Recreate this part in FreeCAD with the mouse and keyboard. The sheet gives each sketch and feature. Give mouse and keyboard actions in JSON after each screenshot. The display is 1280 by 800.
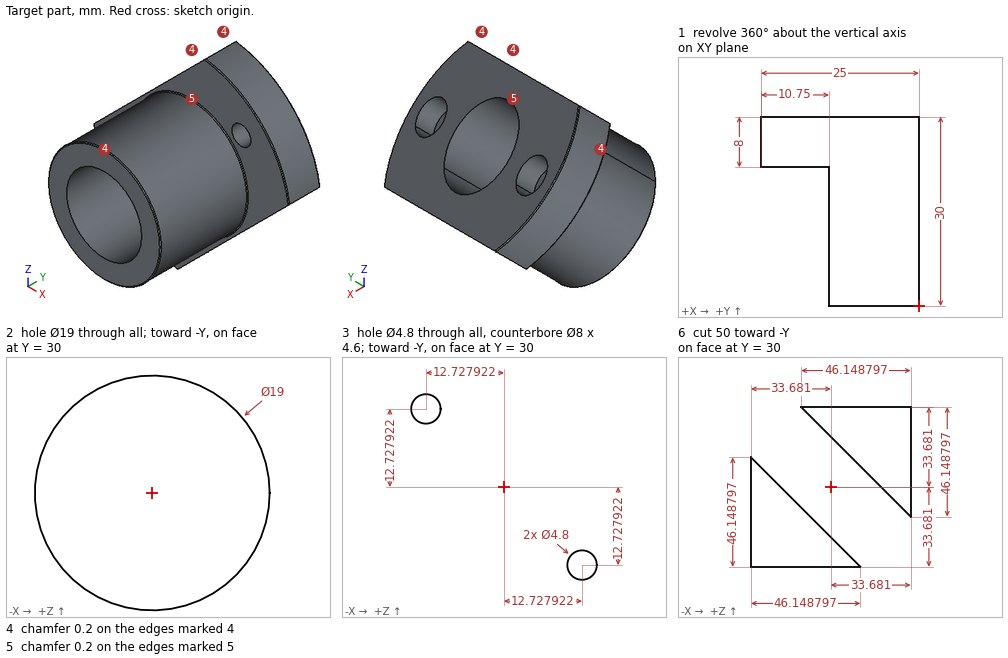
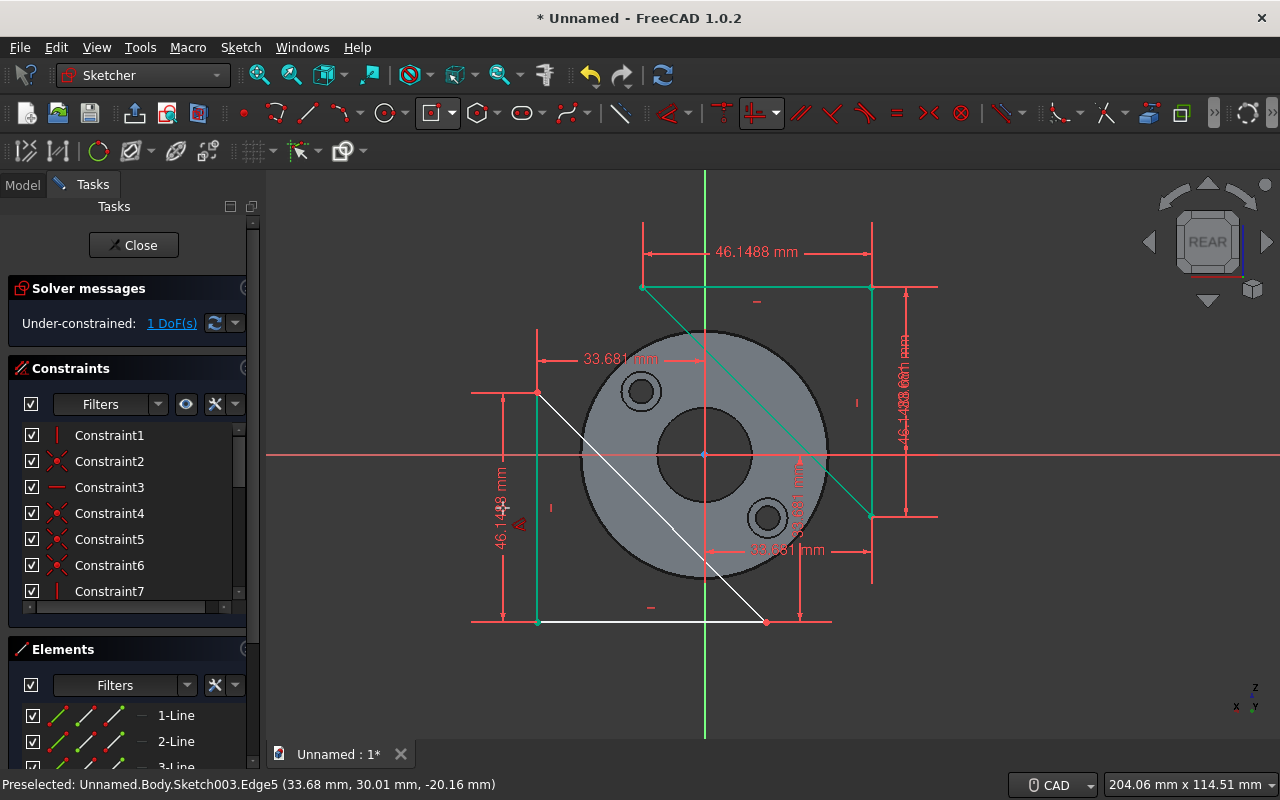
{"action": "left_click", "coordinate": [606, 622]}
{"action": "left_click", "coordinate": [652, 656]}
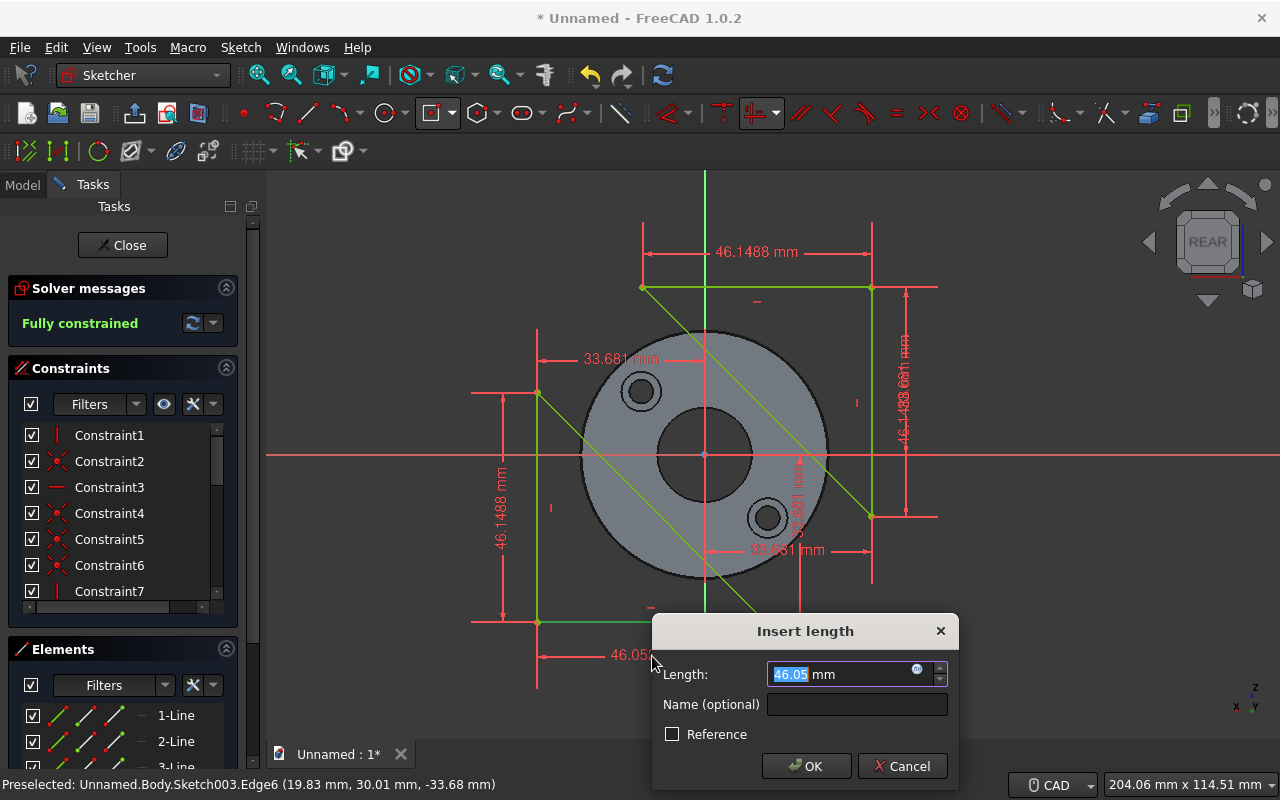
{"action": "type", "text": "46.148797"}
{"action": "key", "text": "Return"}
{"action": "key", "text": "Escape"}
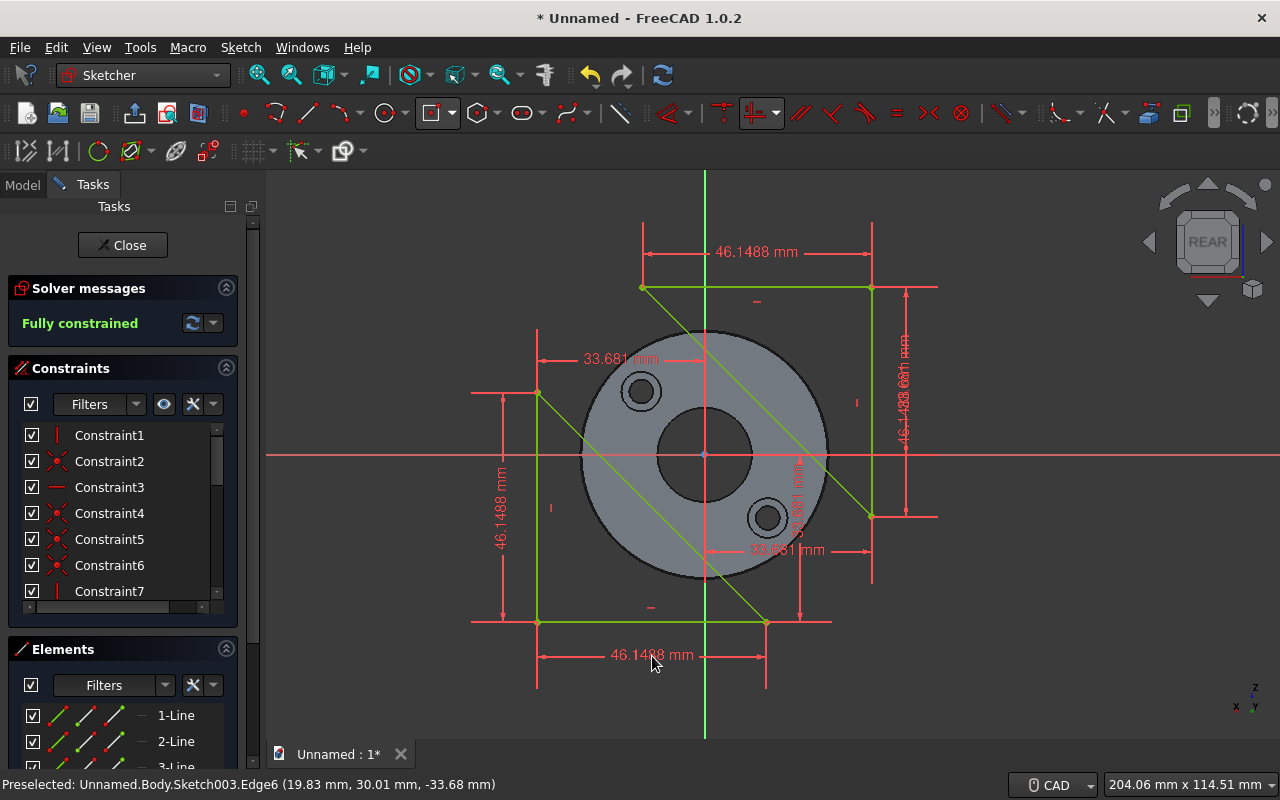
{"action": "left_click", "coordinate": [123, 245]}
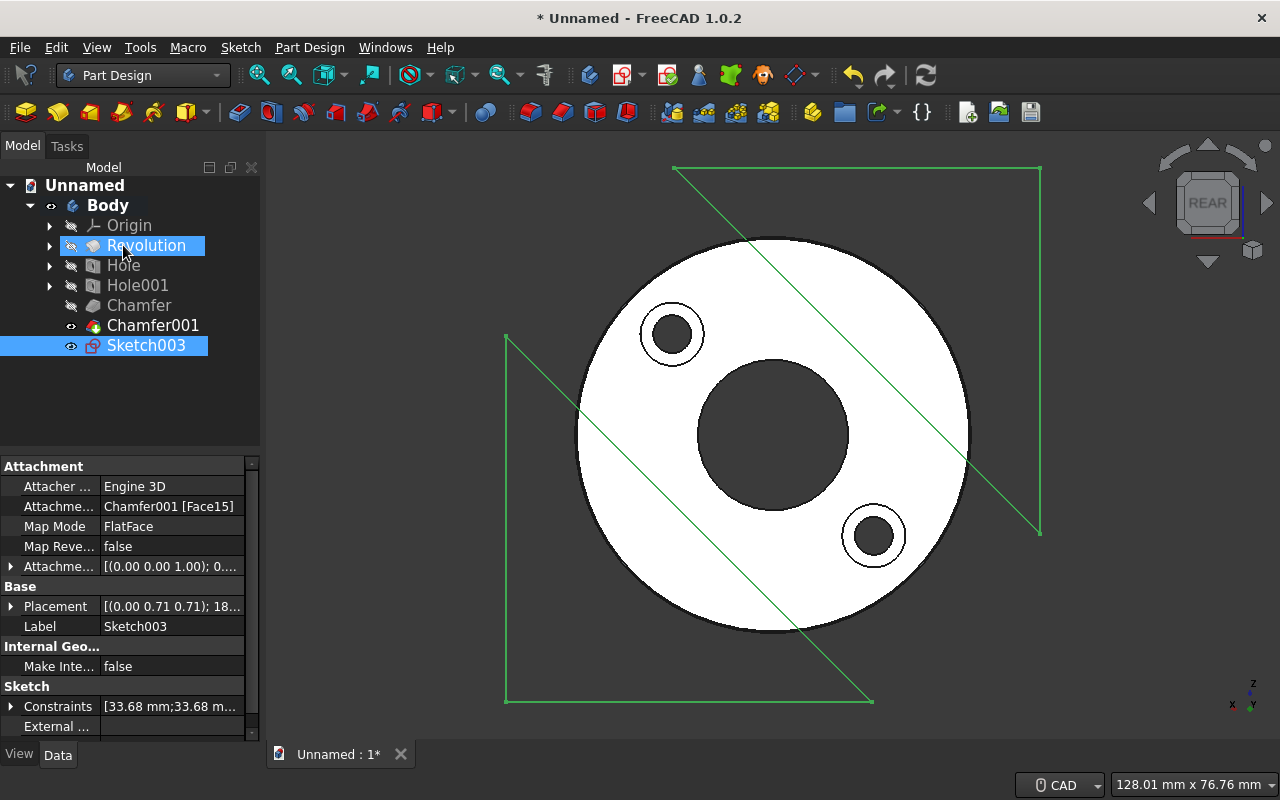
{"action": "left_click", "coordinate": [240, 112]}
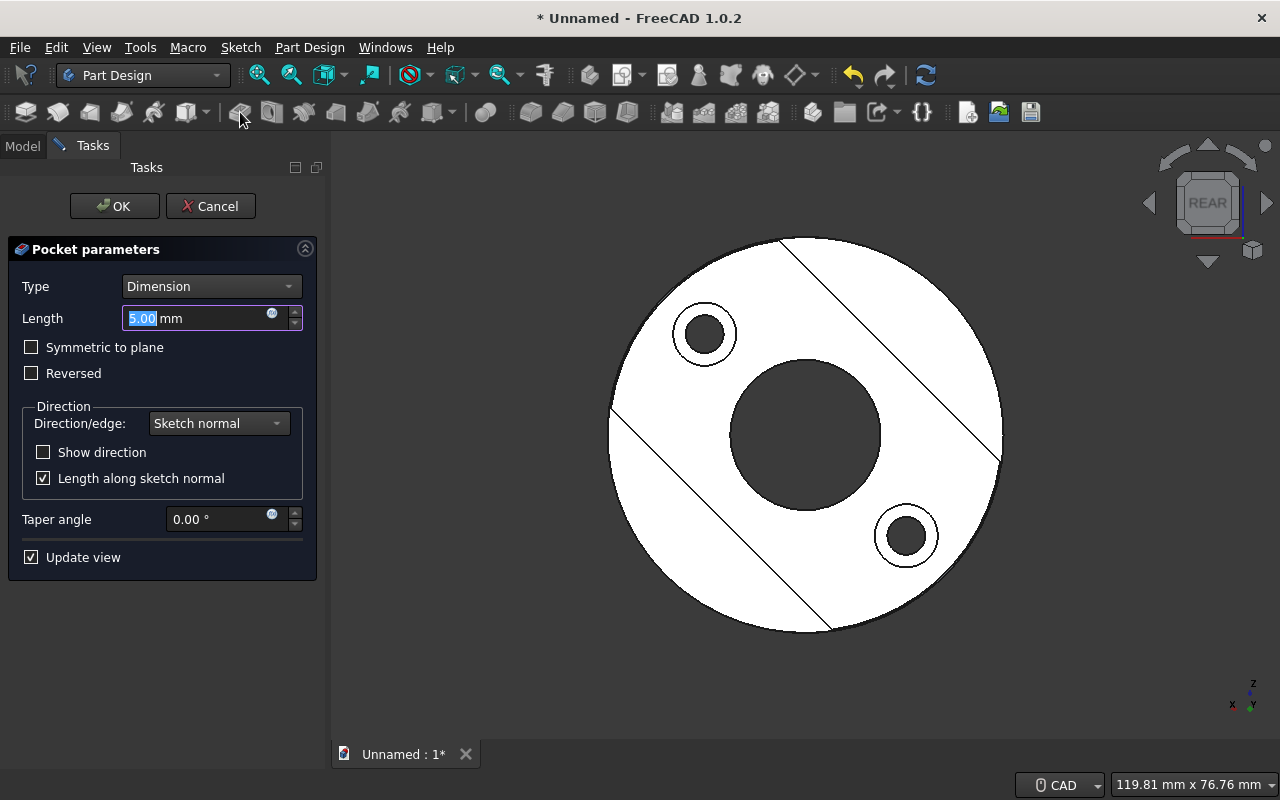
{"action": "type", "text": "50"}
{"action": "key", "text": "Tab"}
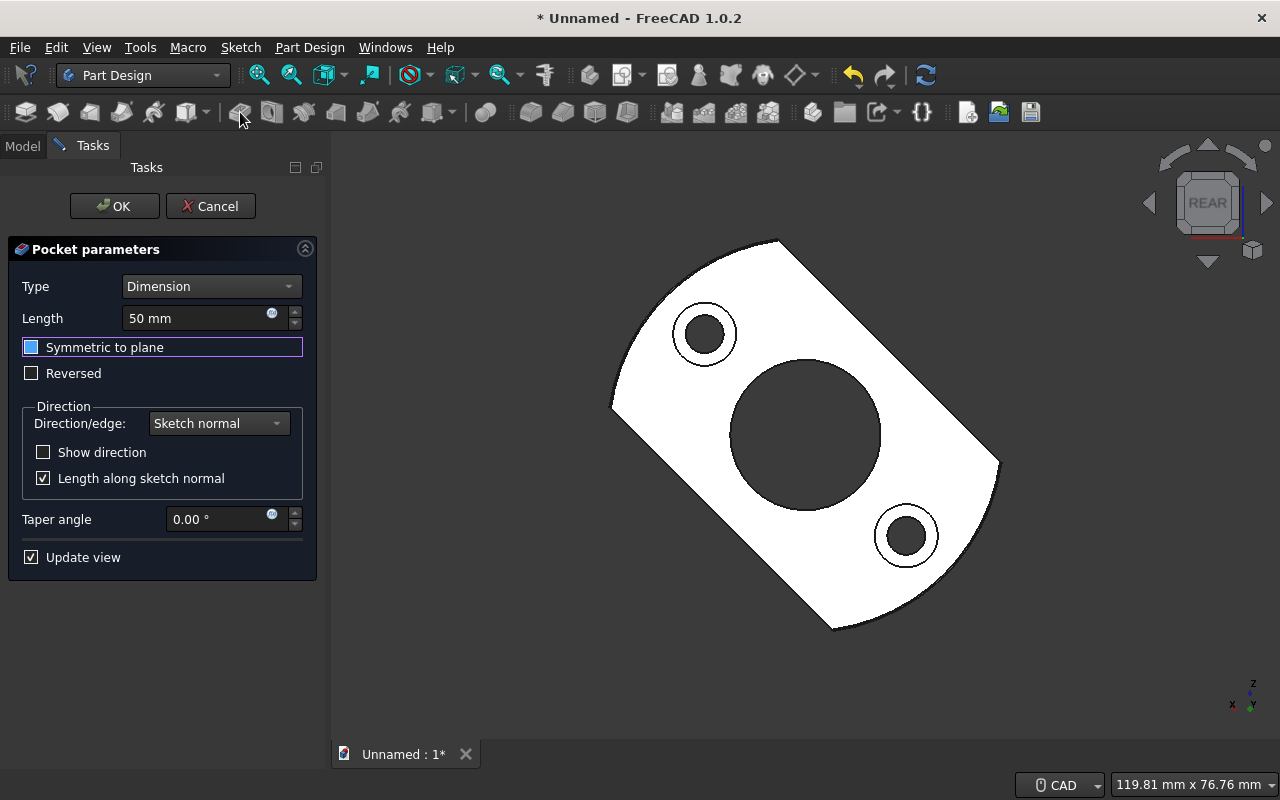
{"action": "left_click", "coordinate": [115, 206]}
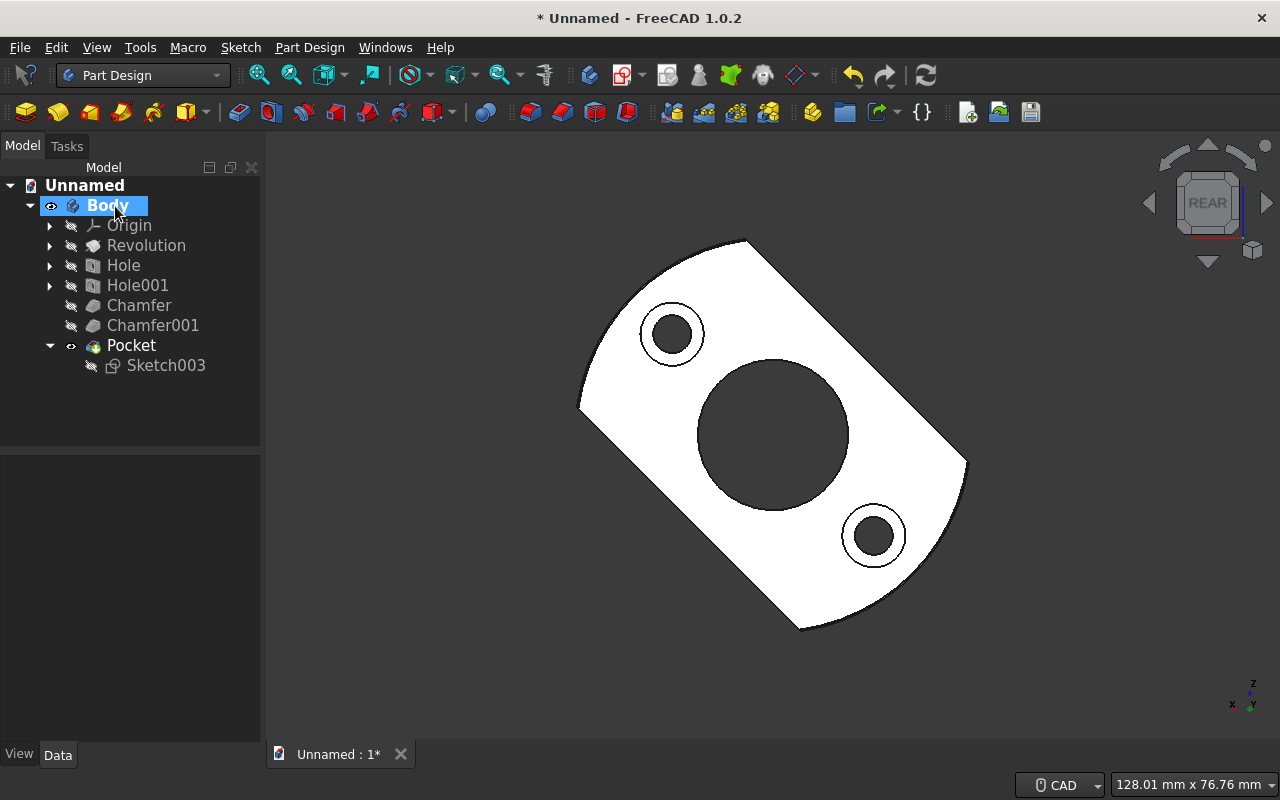
{"action": "key", "text": "0"}